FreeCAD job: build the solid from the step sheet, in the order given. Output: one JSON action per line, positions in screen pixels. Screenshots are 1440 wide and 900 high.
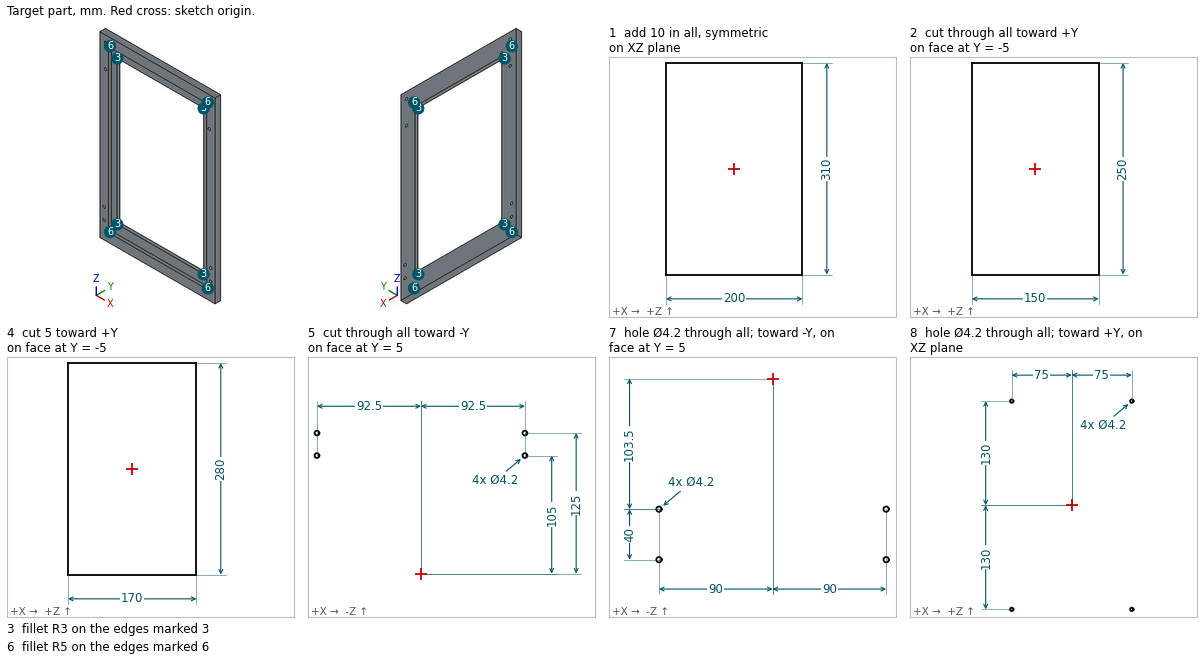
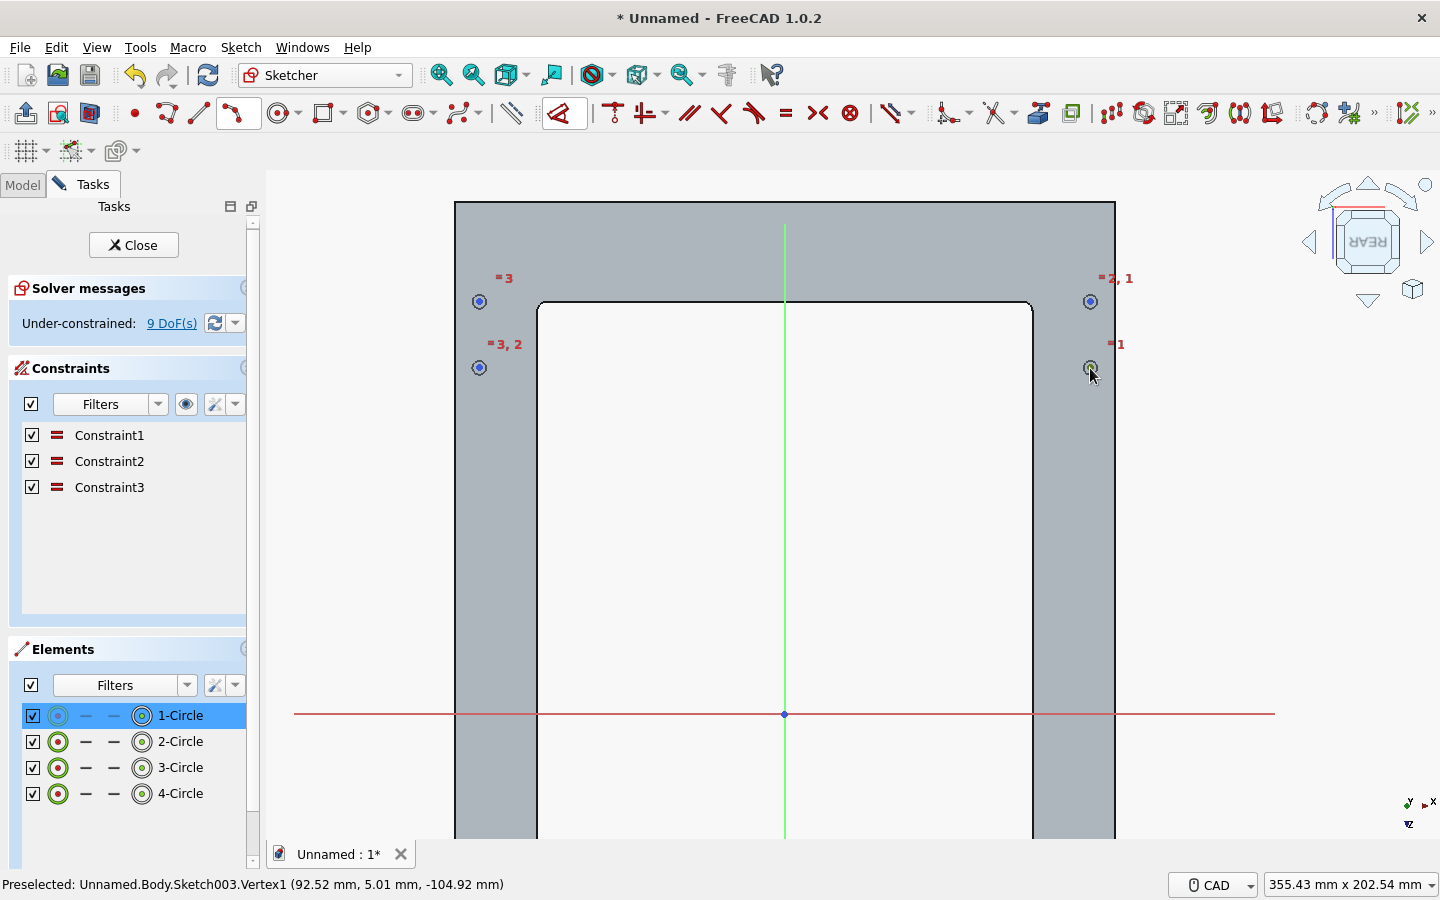
{"action": "left_click", "coordinate": [1090, 302]}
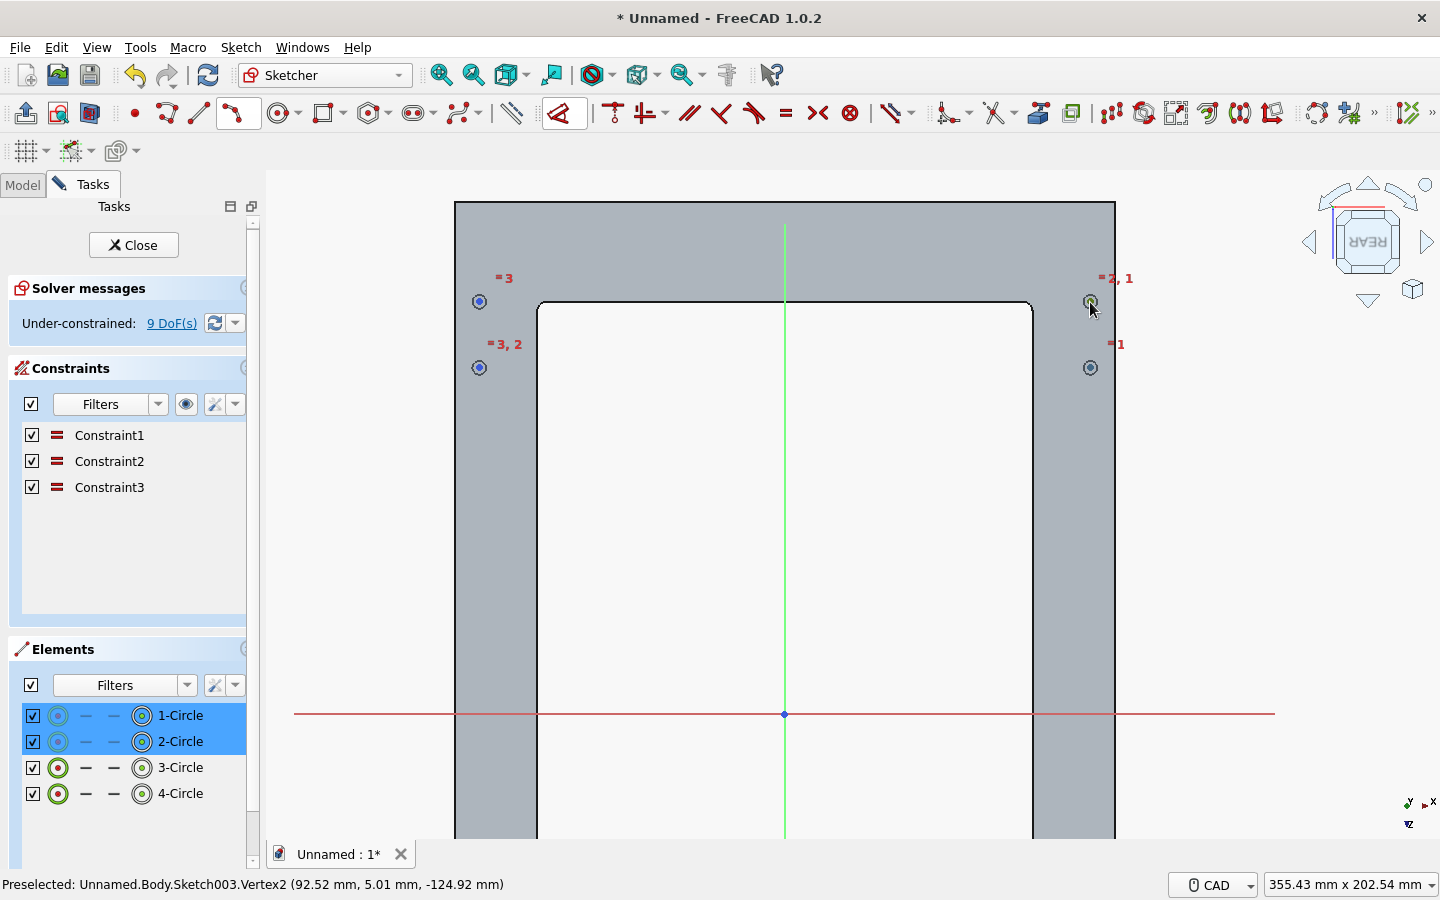
{"action": "key", "text": "v"}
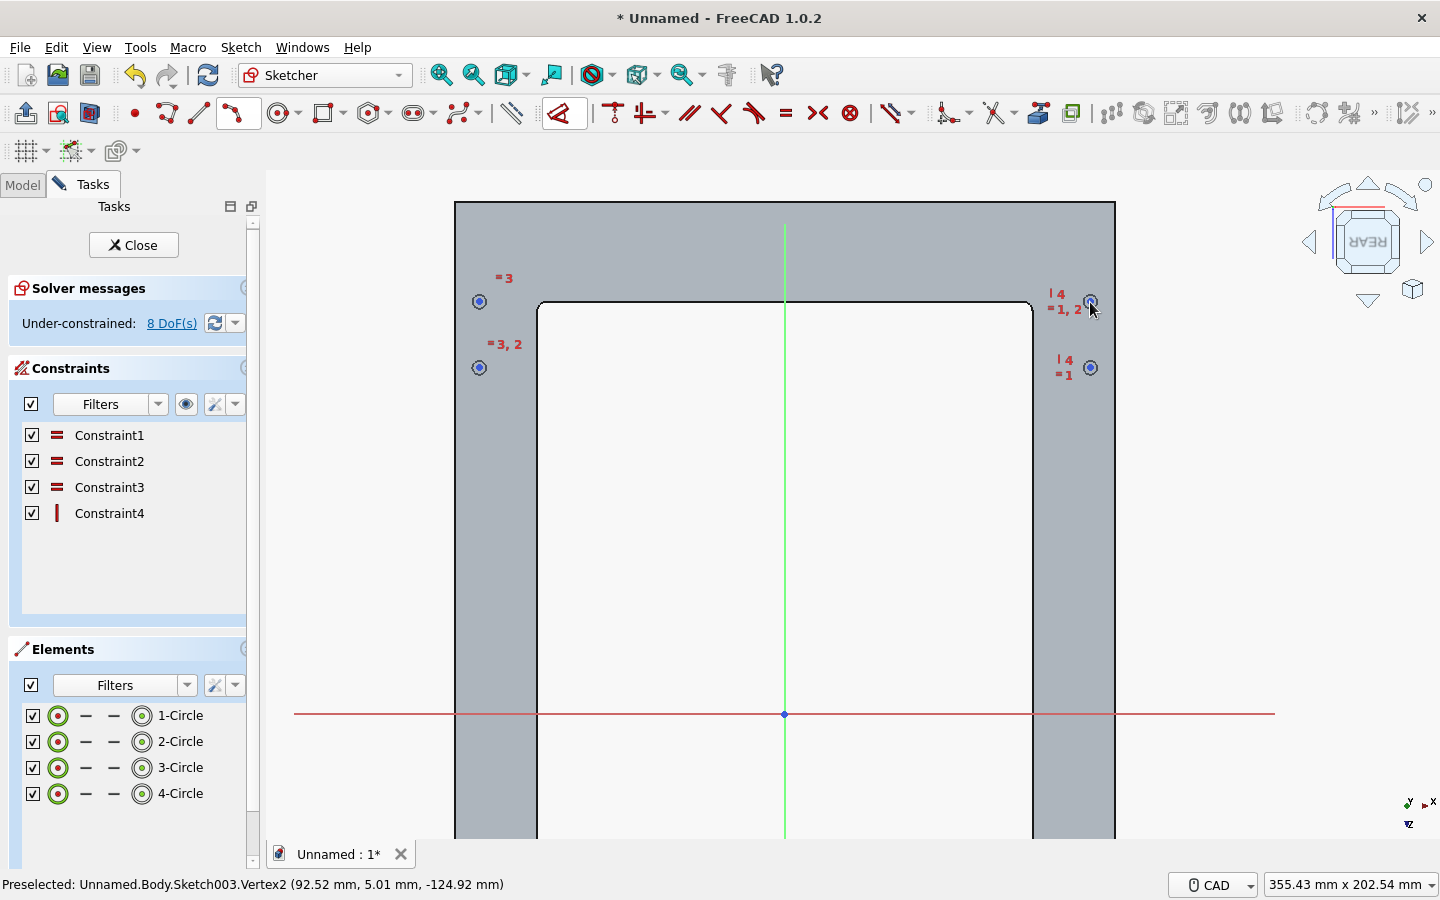
{"action": "left_click", "coordinate": [1090, 368]}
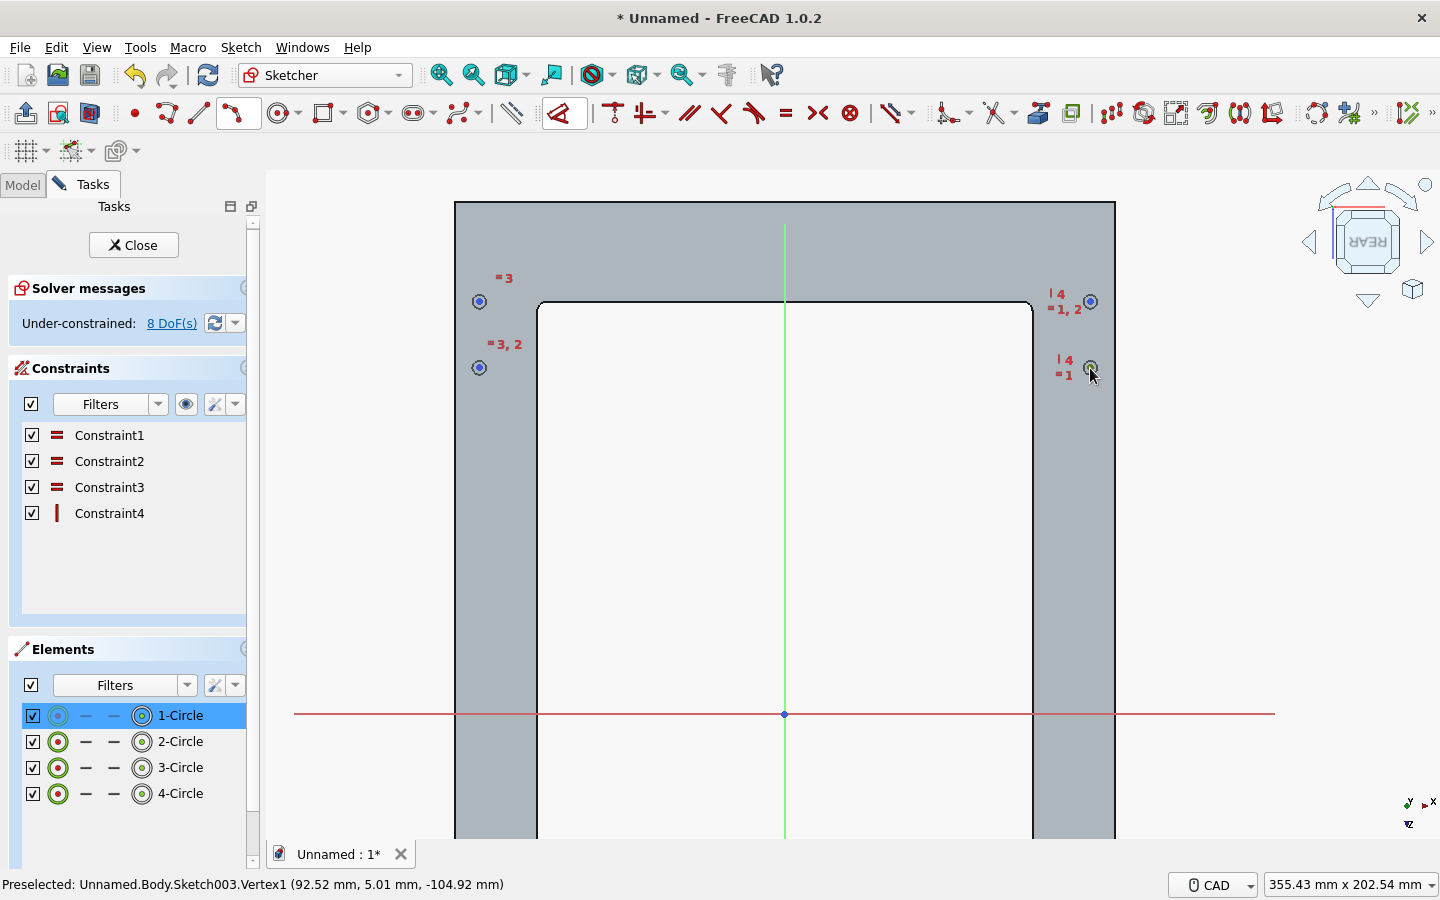
{"action": "left_click", "coordinate": [479, 368]}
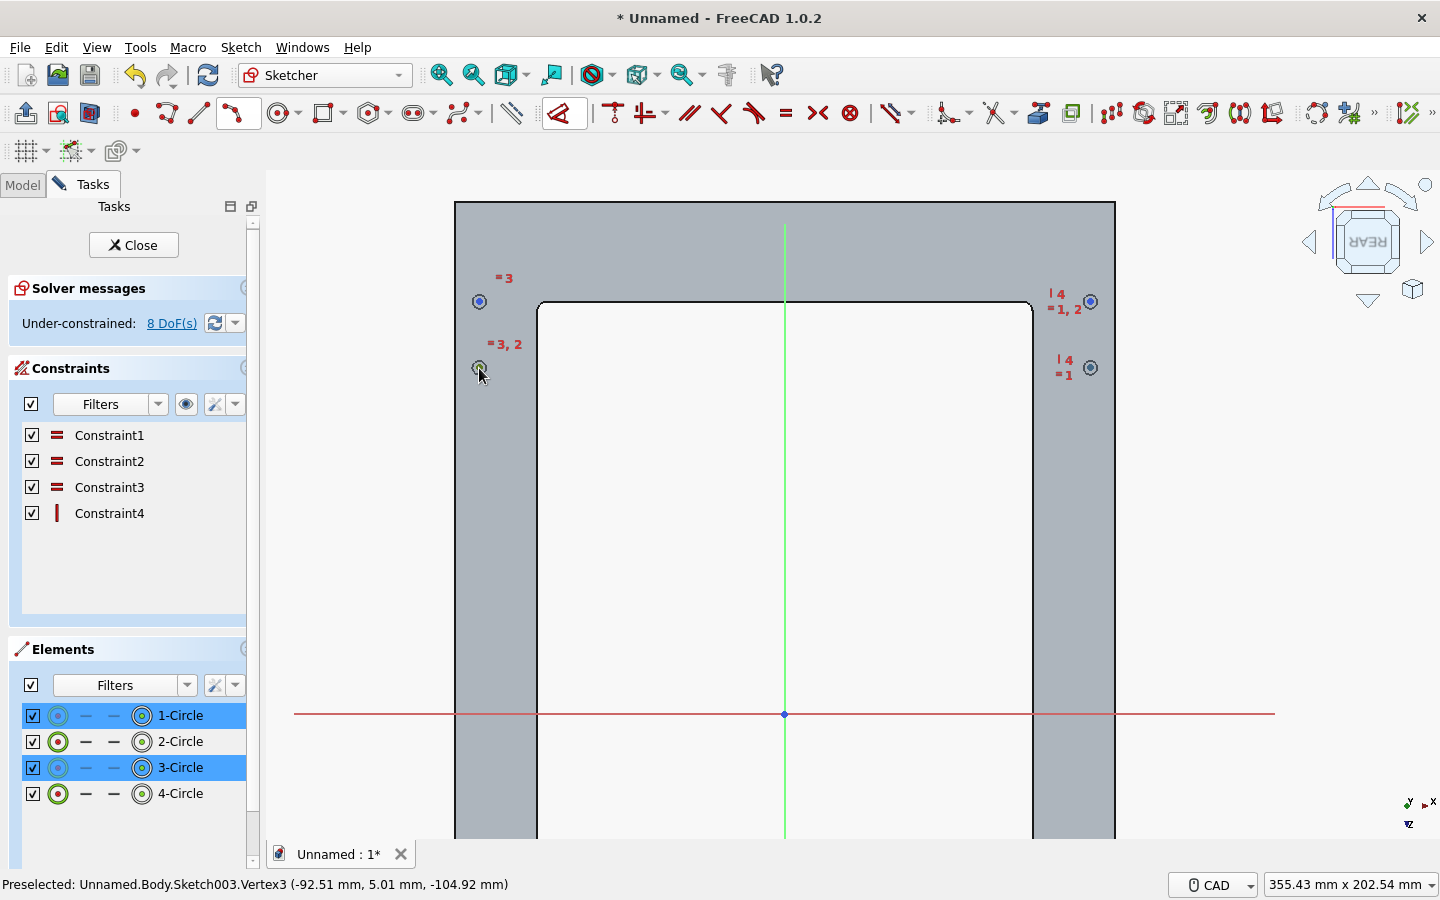
{"action": "left_click", "coordinate": [668, 114]}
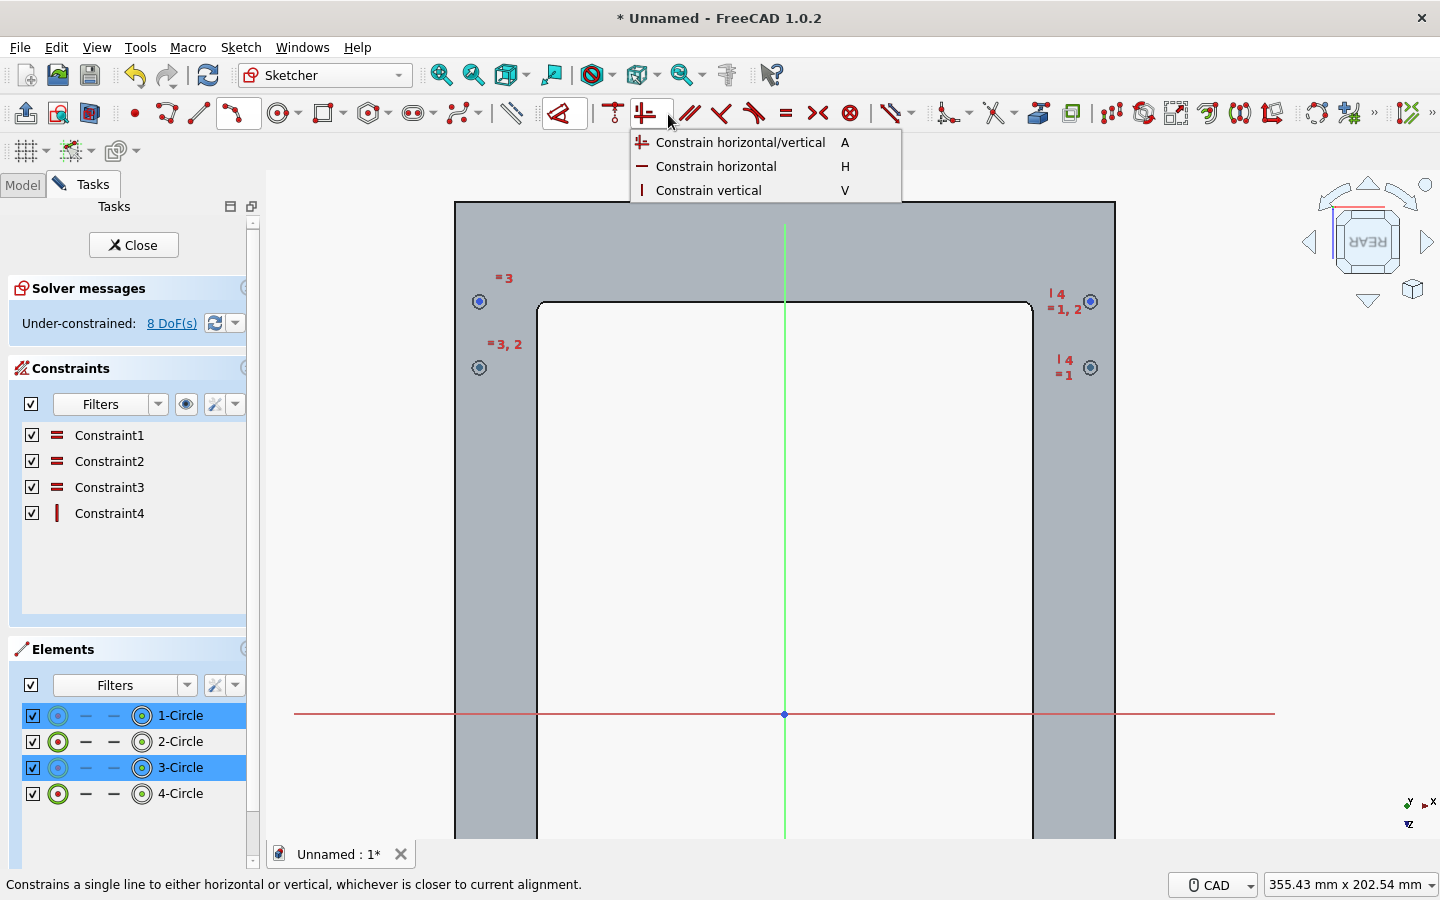
{"action": "left_click", "coordinate": [766, 166]}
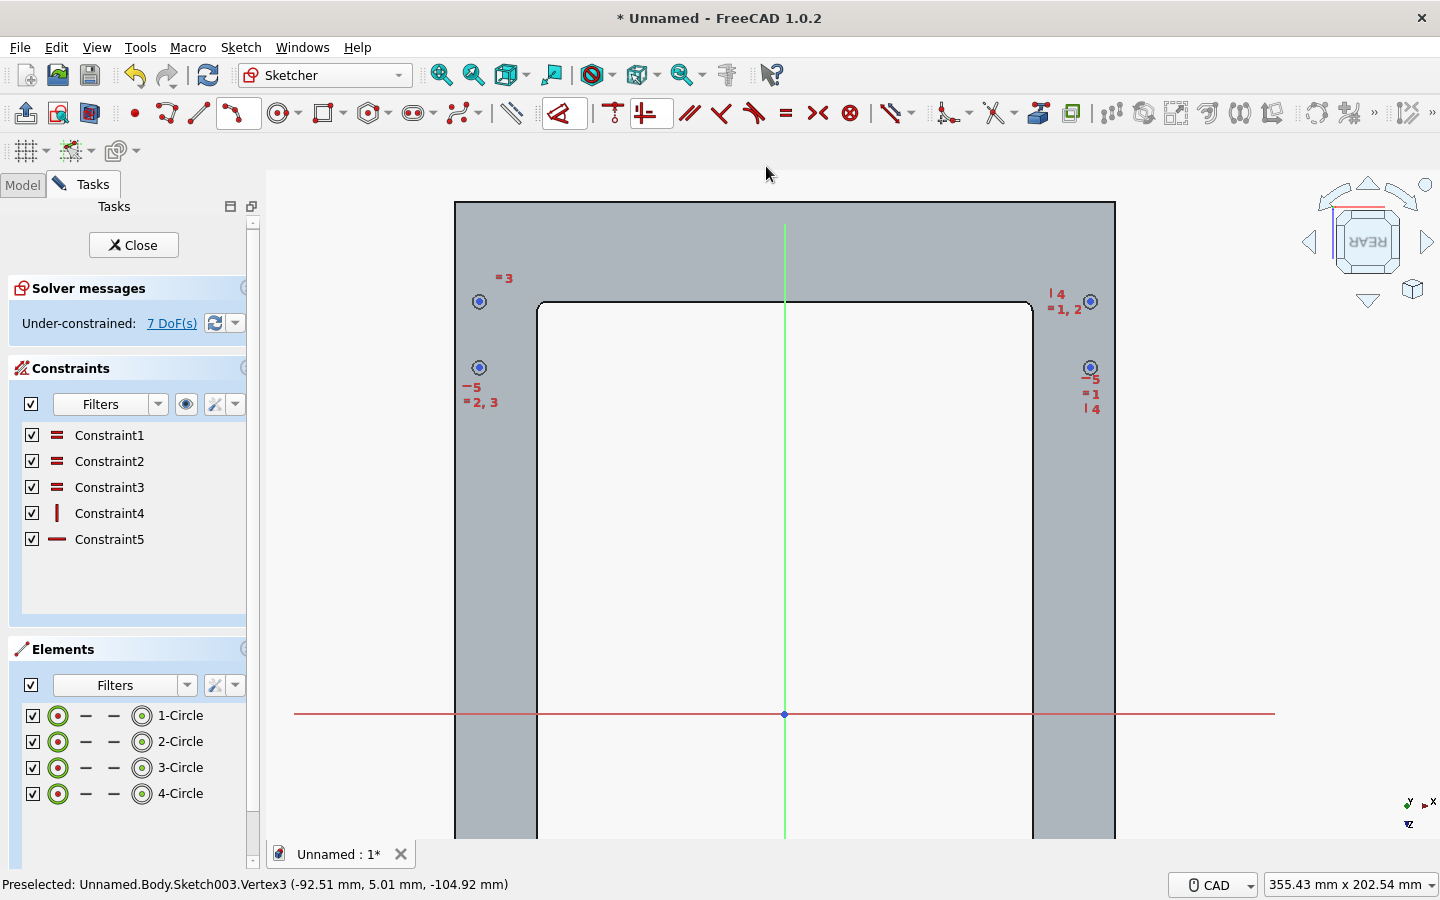
{"action": "left_click", "coordinate": [479, 368]}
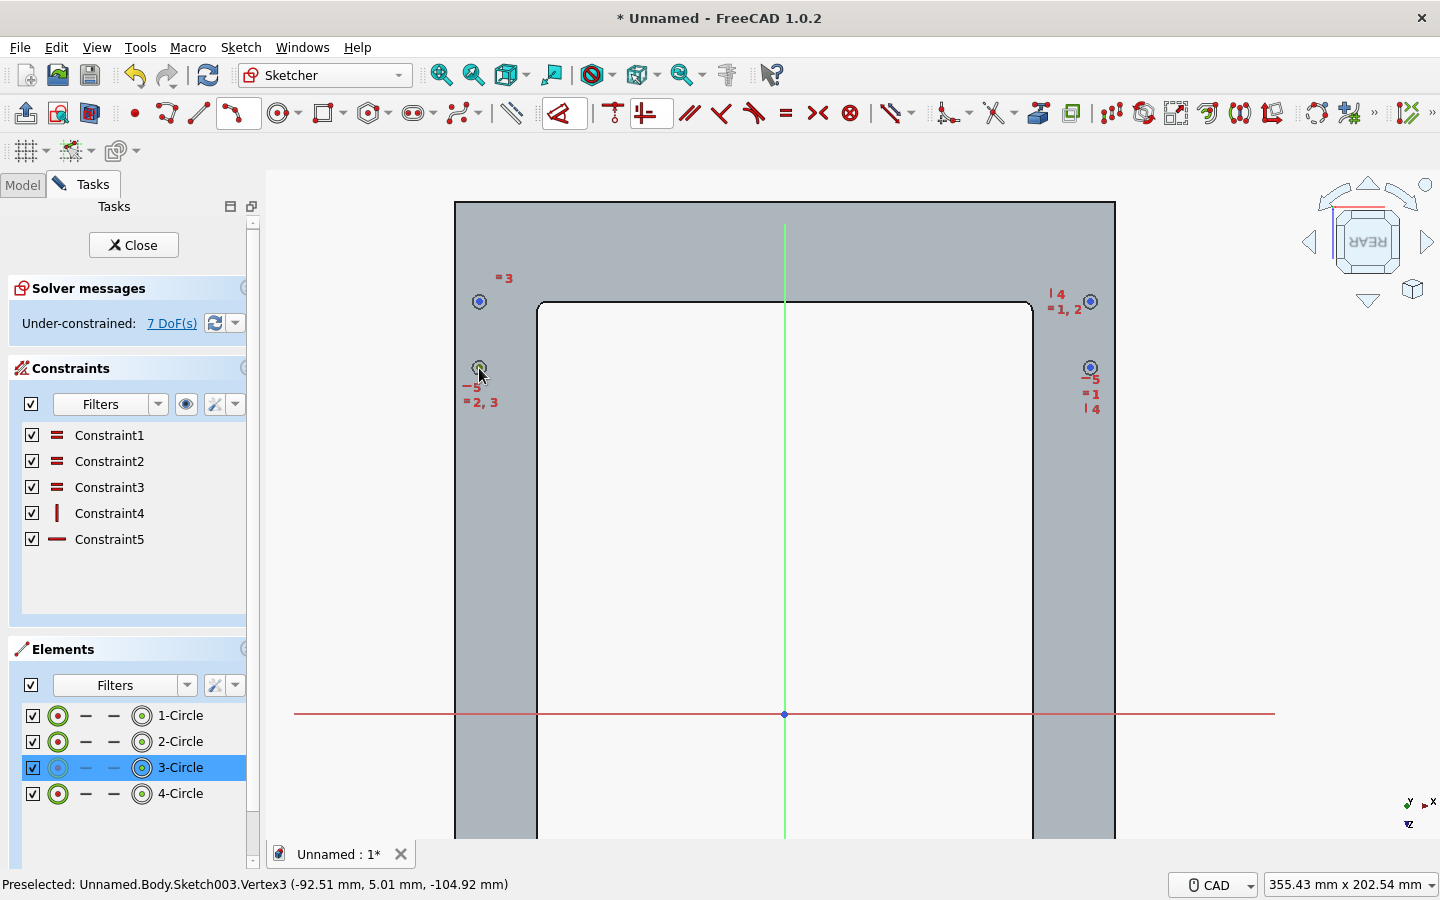
{"action": "left_click", "coordinate": [479, 302]}